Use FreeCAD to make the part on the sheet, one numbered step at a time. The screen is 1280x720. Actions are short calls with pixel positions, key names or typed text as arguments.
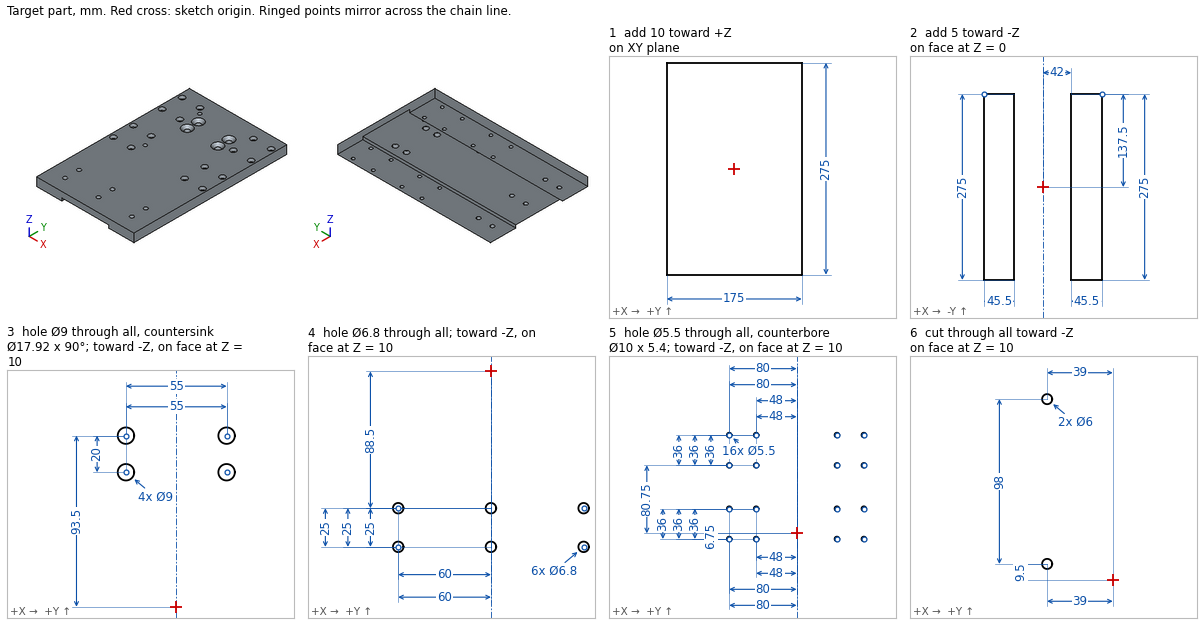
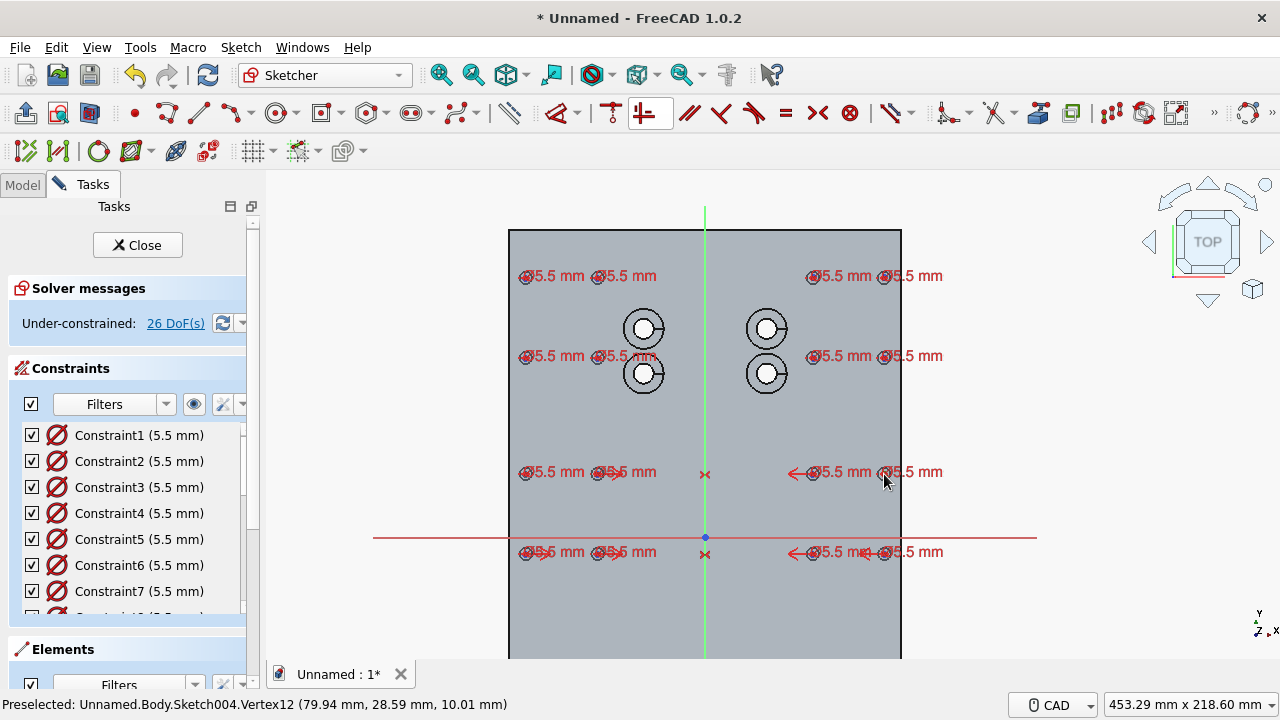
click(705, 600)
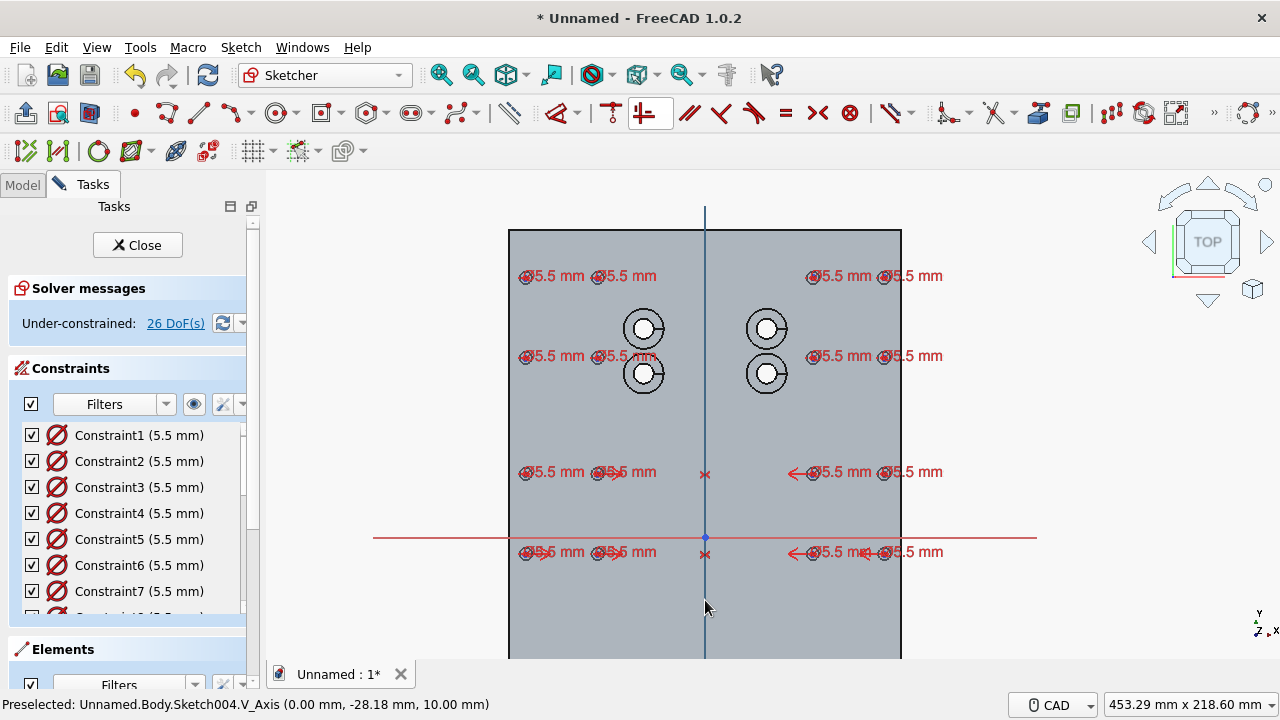
click(818, 114)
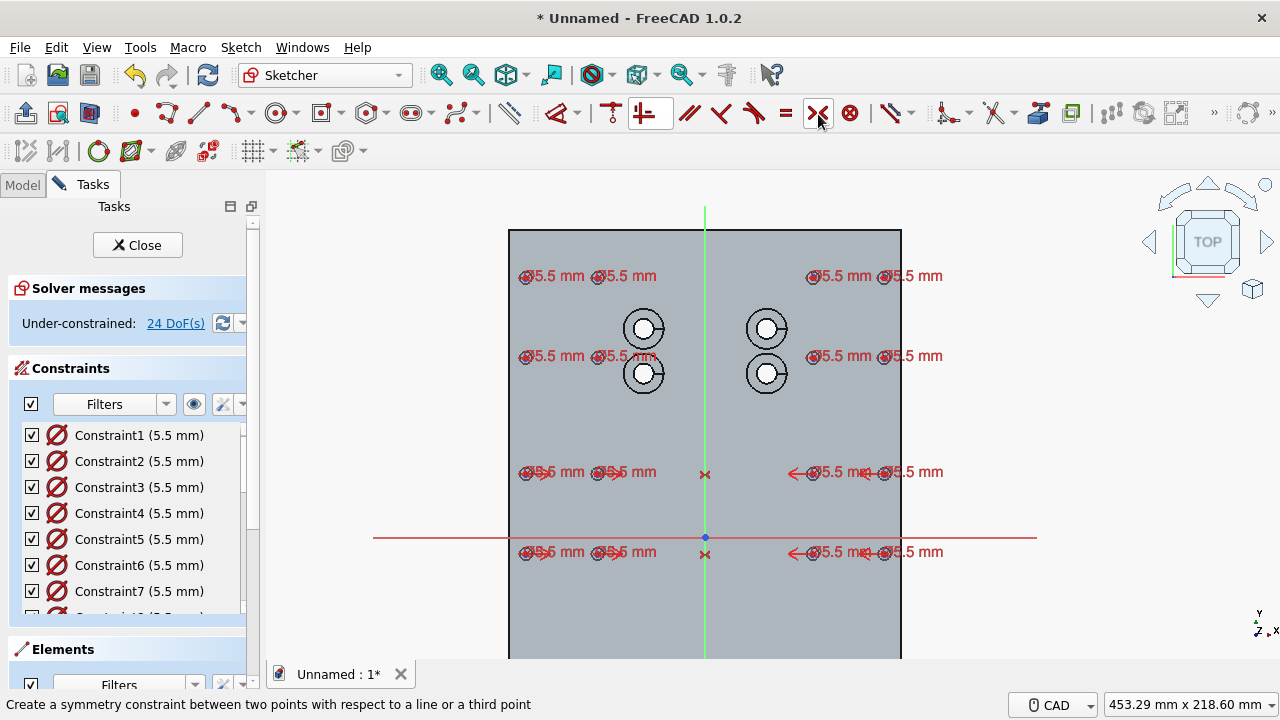
click(598, 358)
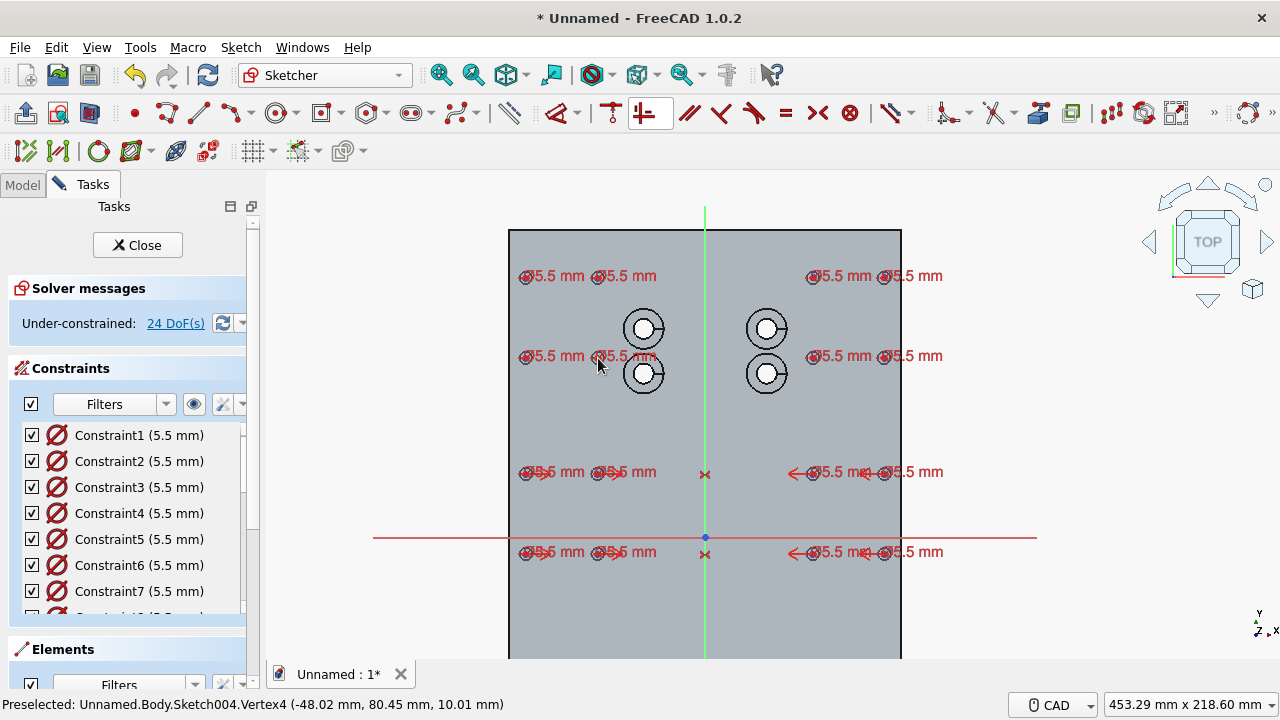
click(813, 358)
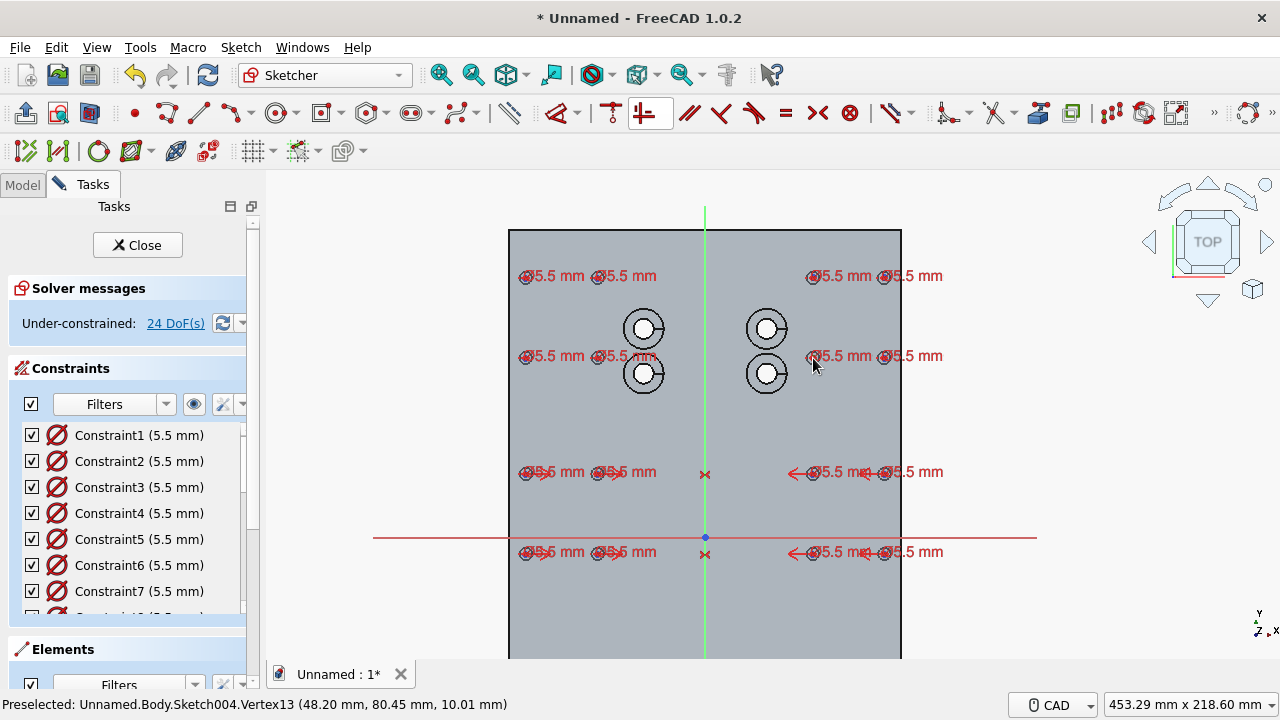
click(705, 600)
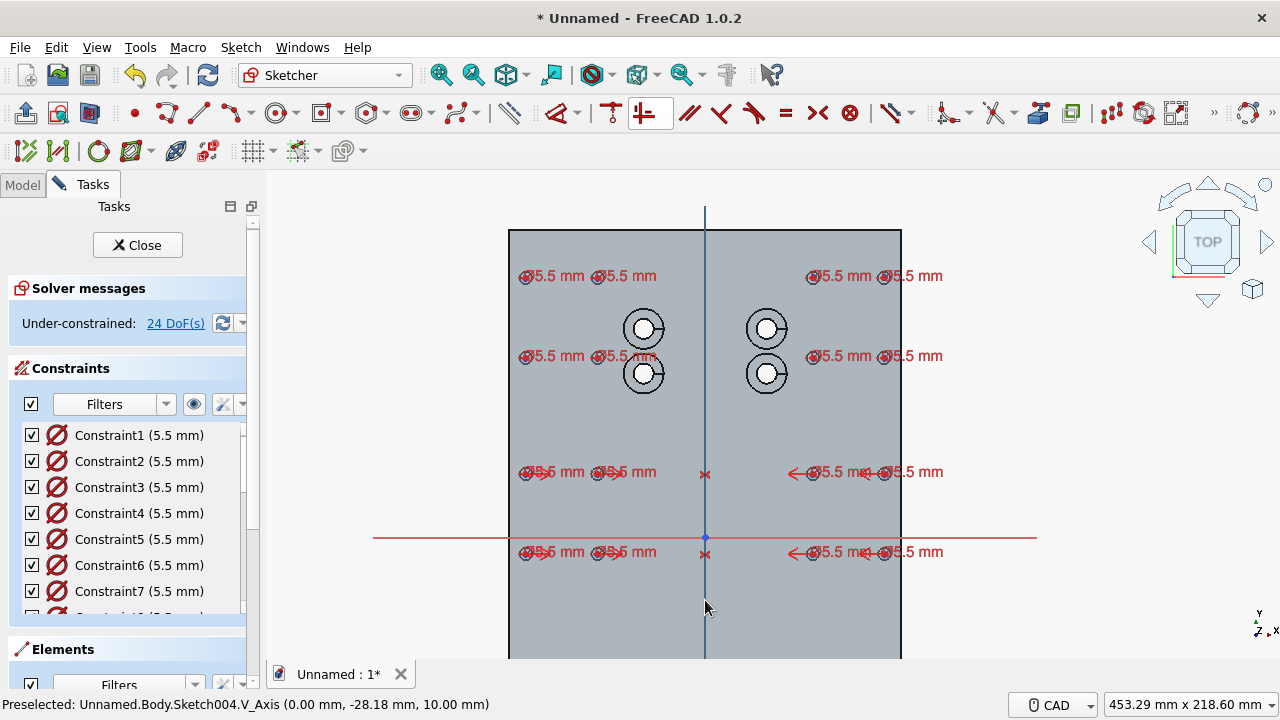
key(s)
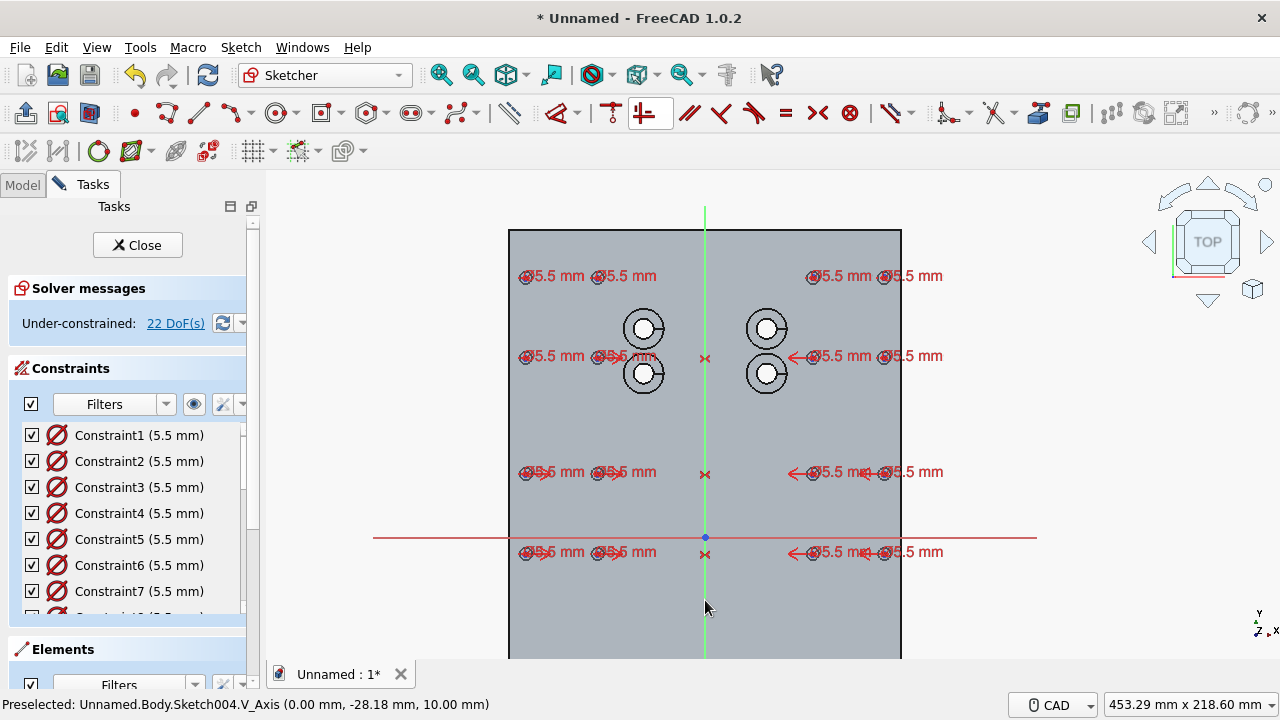
click(526, 358)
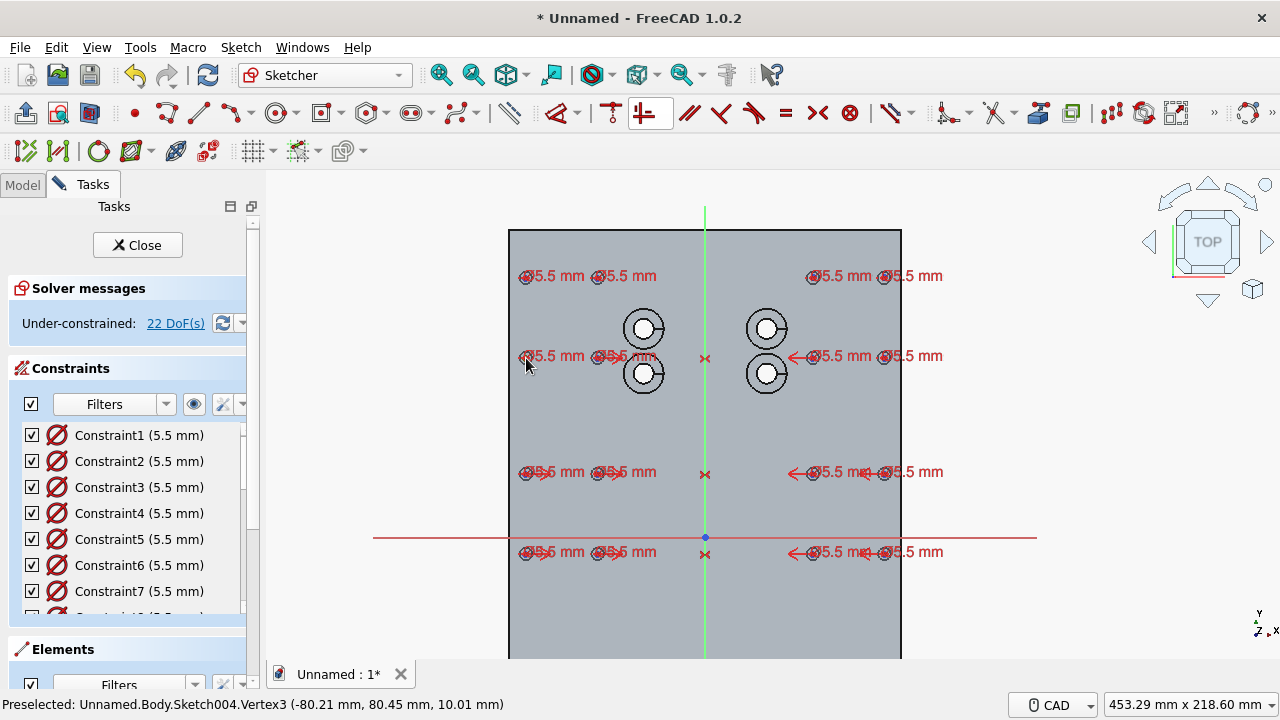
click(884, 358)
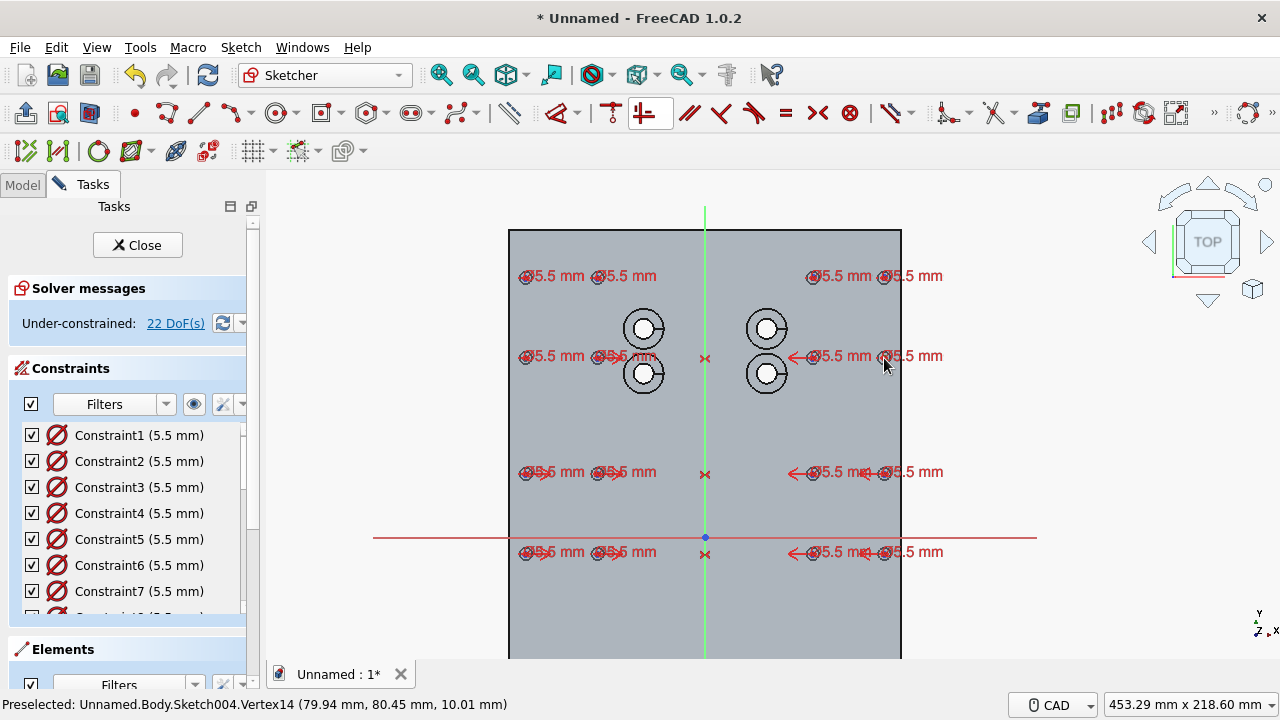
click(705, 600)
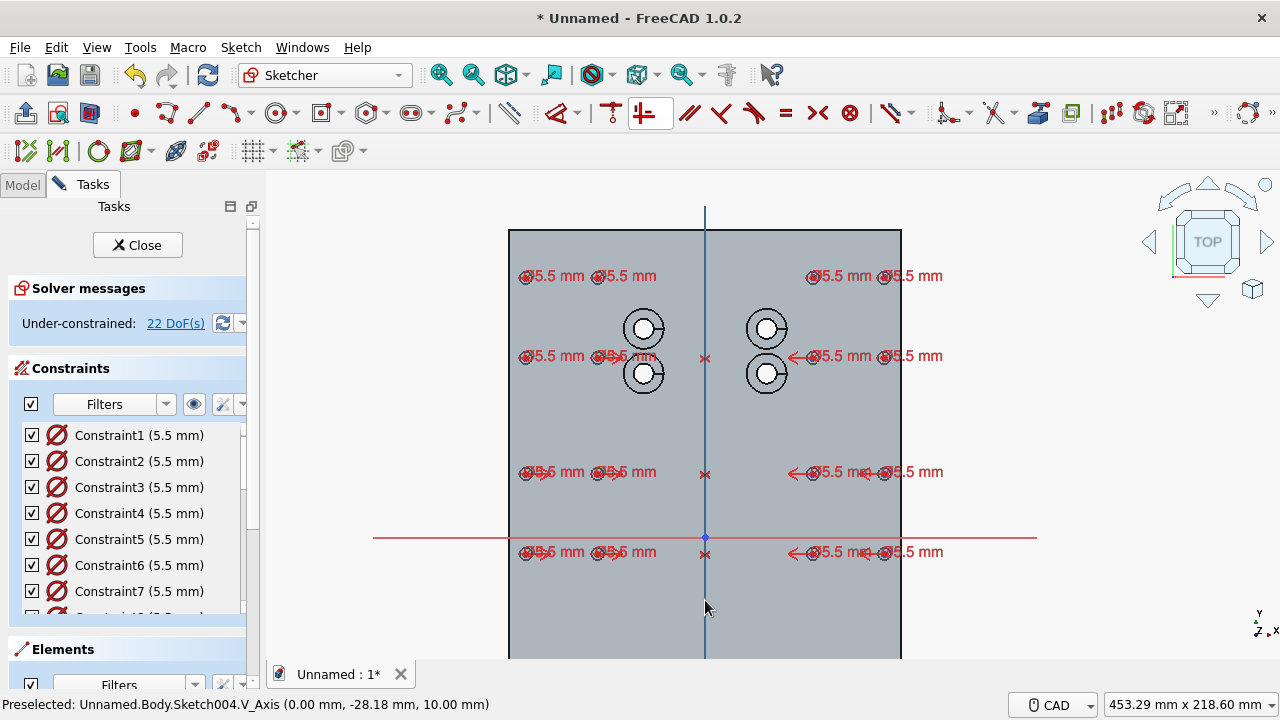
key(s)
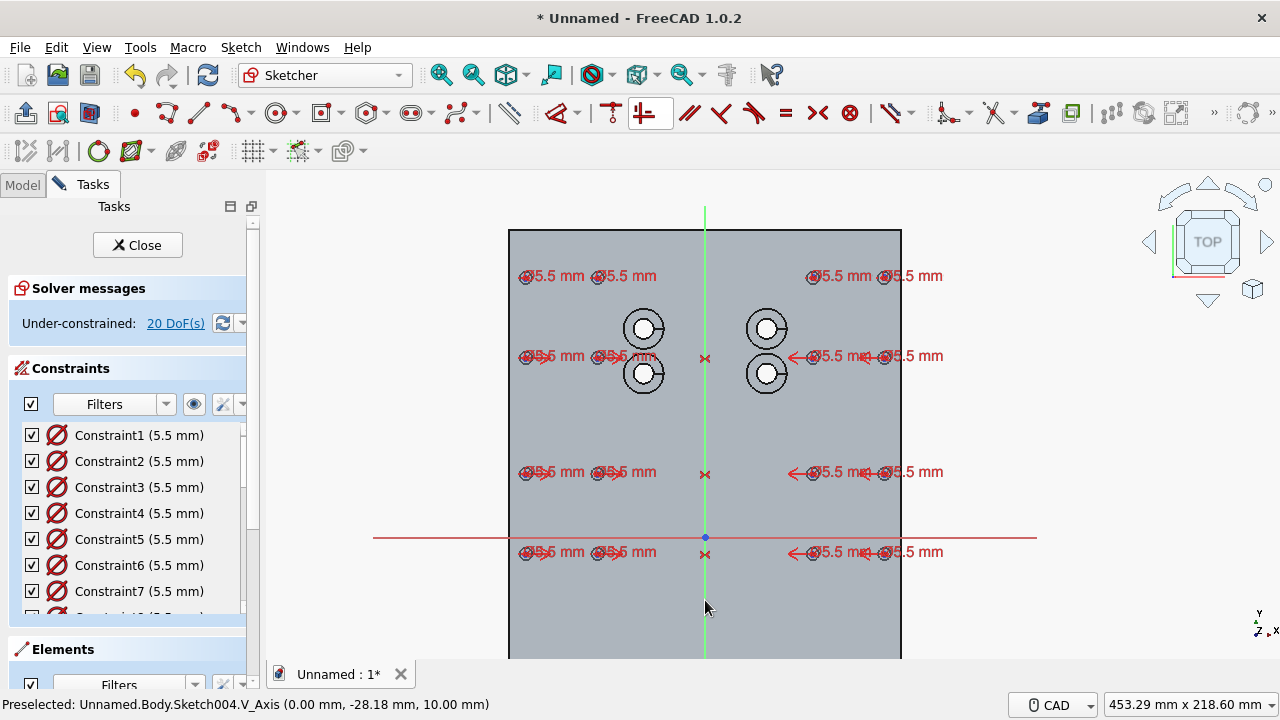
click(598, 278)